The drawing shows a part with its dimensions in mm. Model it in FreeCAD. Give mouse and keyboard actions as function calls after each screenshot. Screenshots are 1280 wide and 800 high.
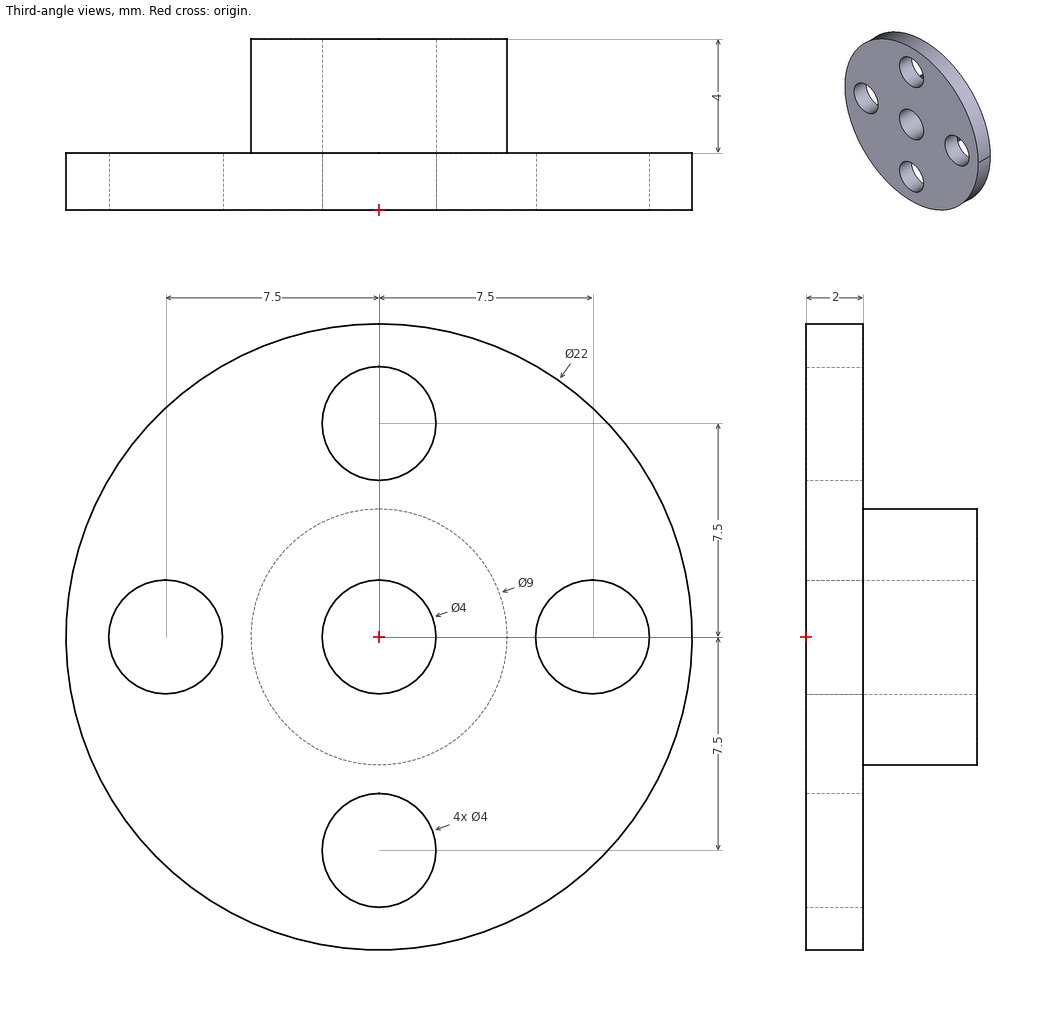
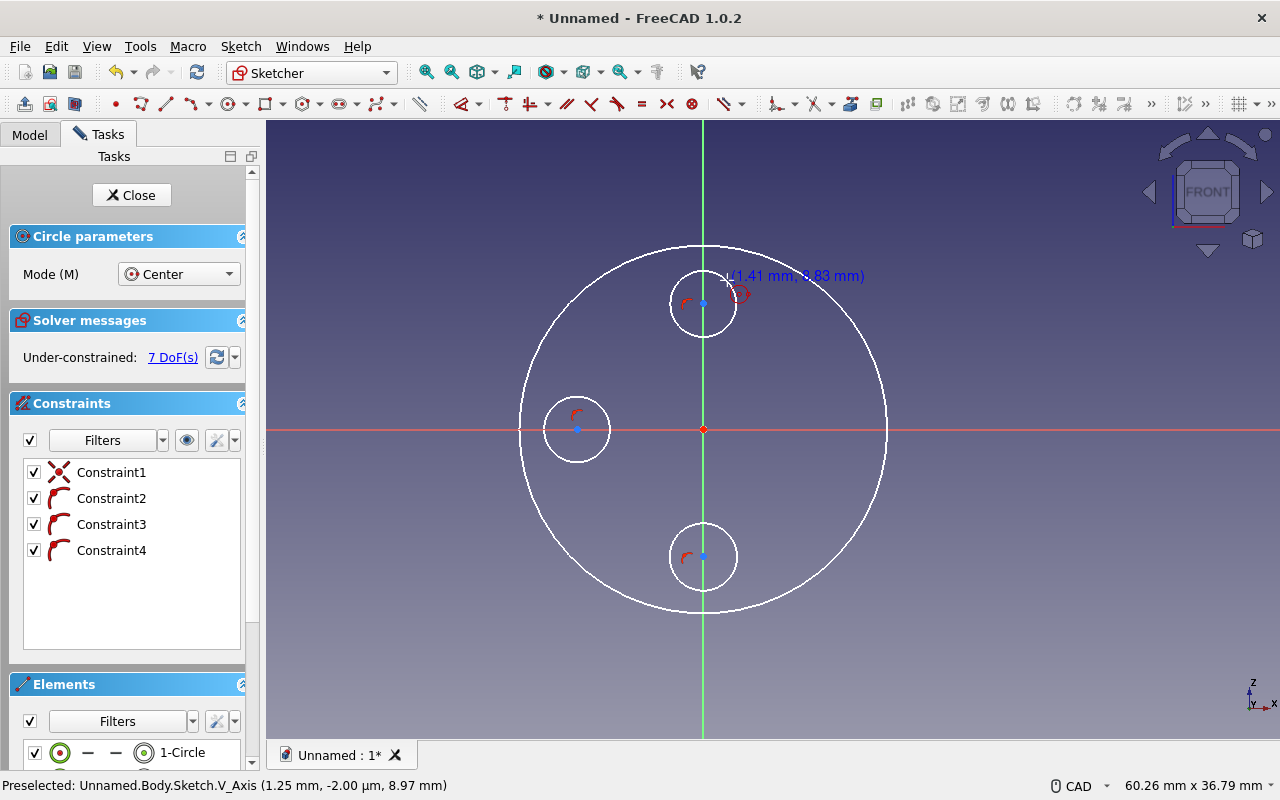
click(830, 430)
click(853, 406)
key(Escape)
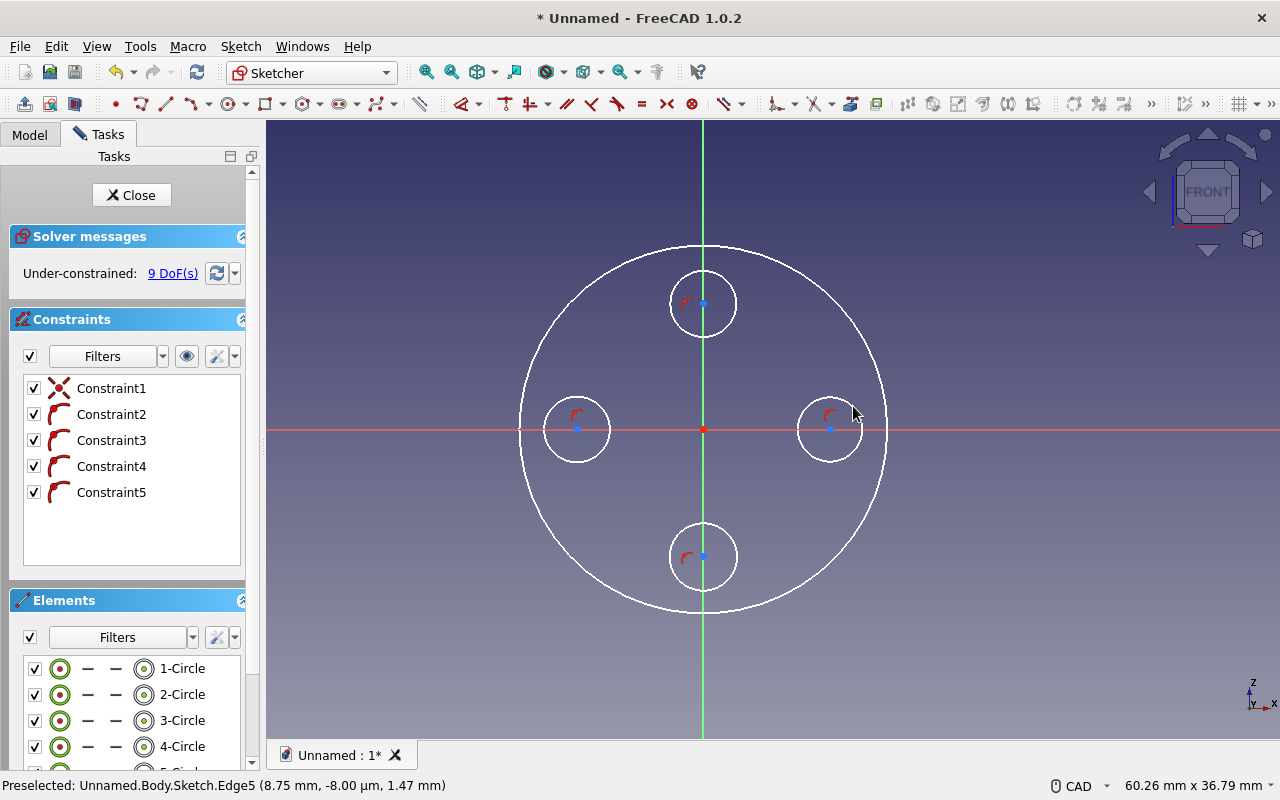
click(727, 533)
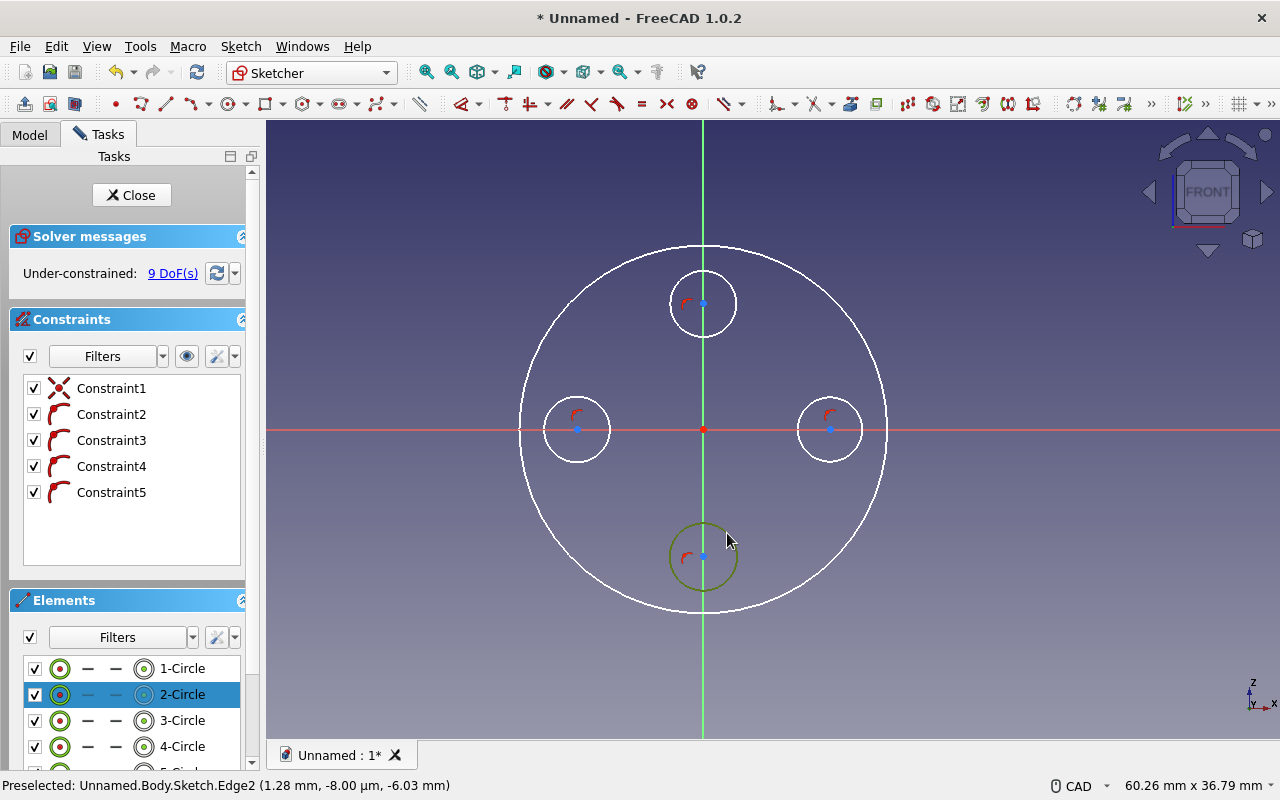
click(600, 406)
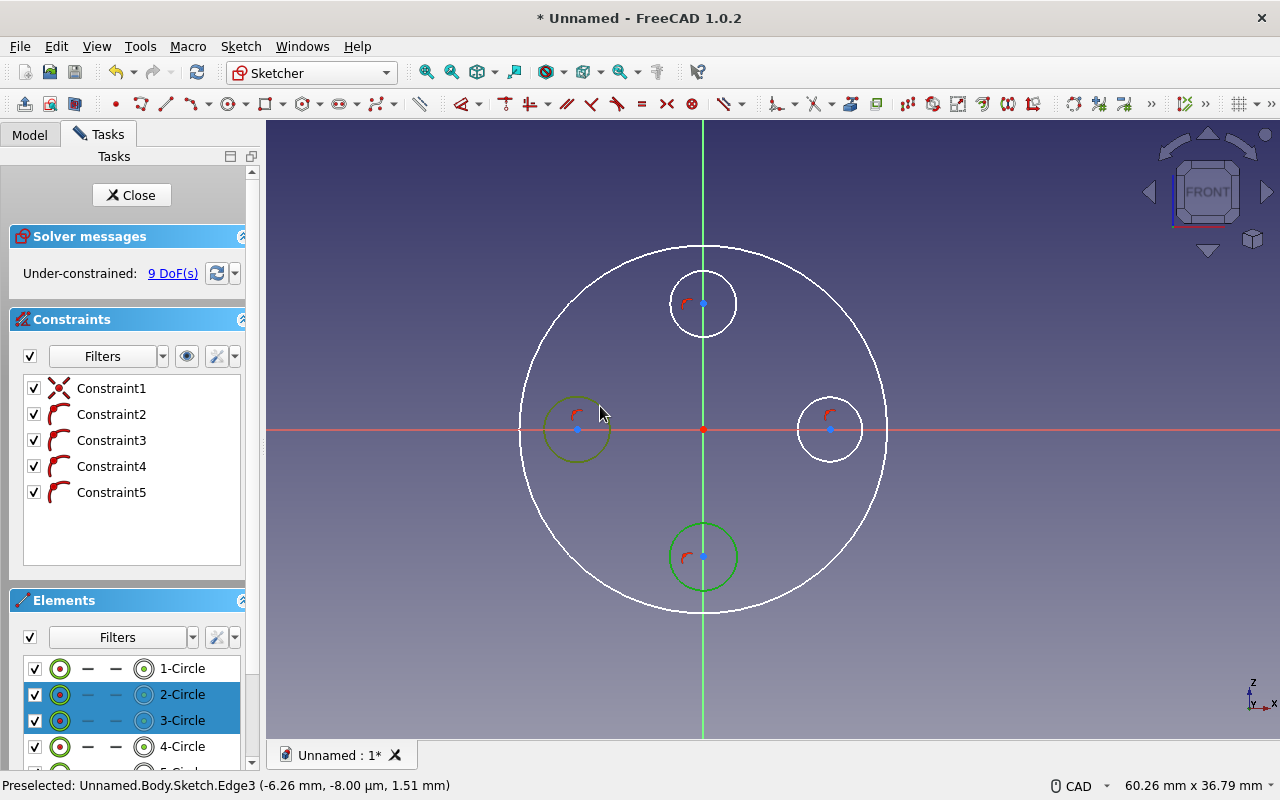
click(727, 281)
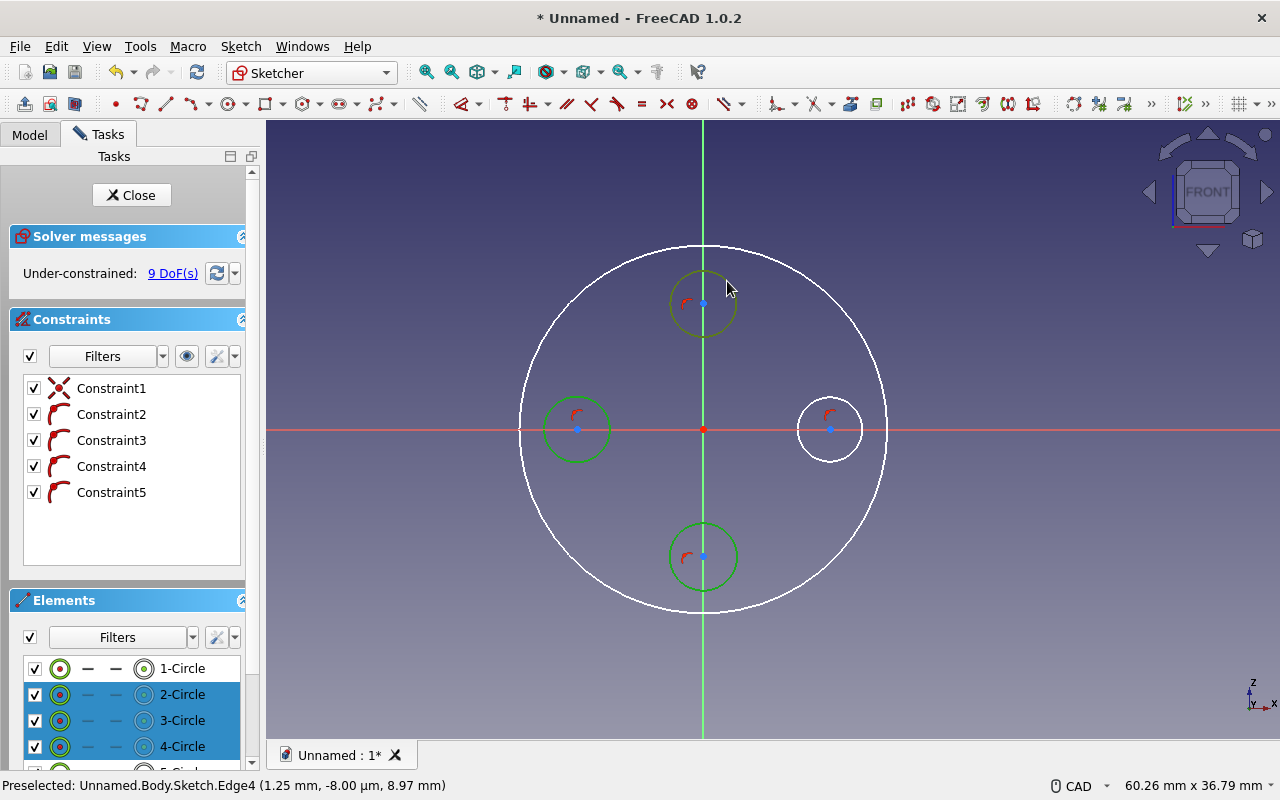
click(853, 407)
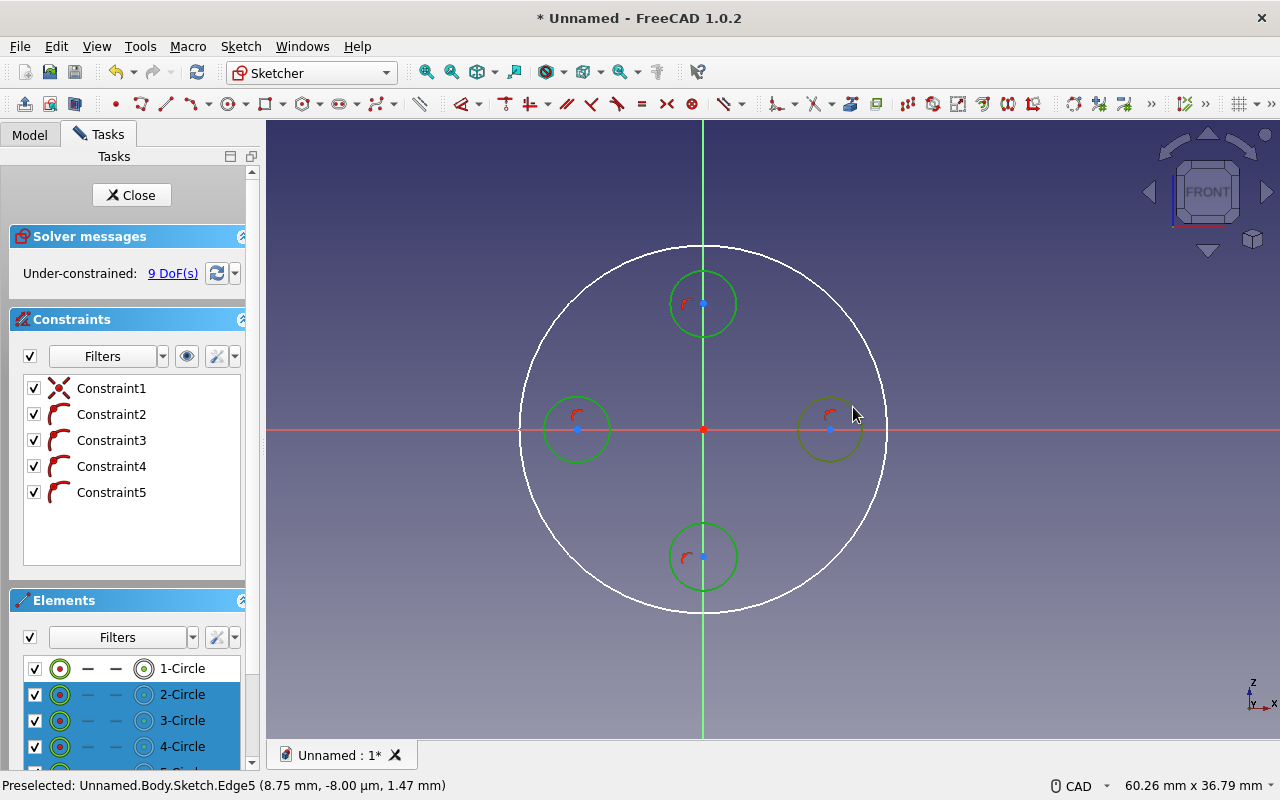
click(642, 104)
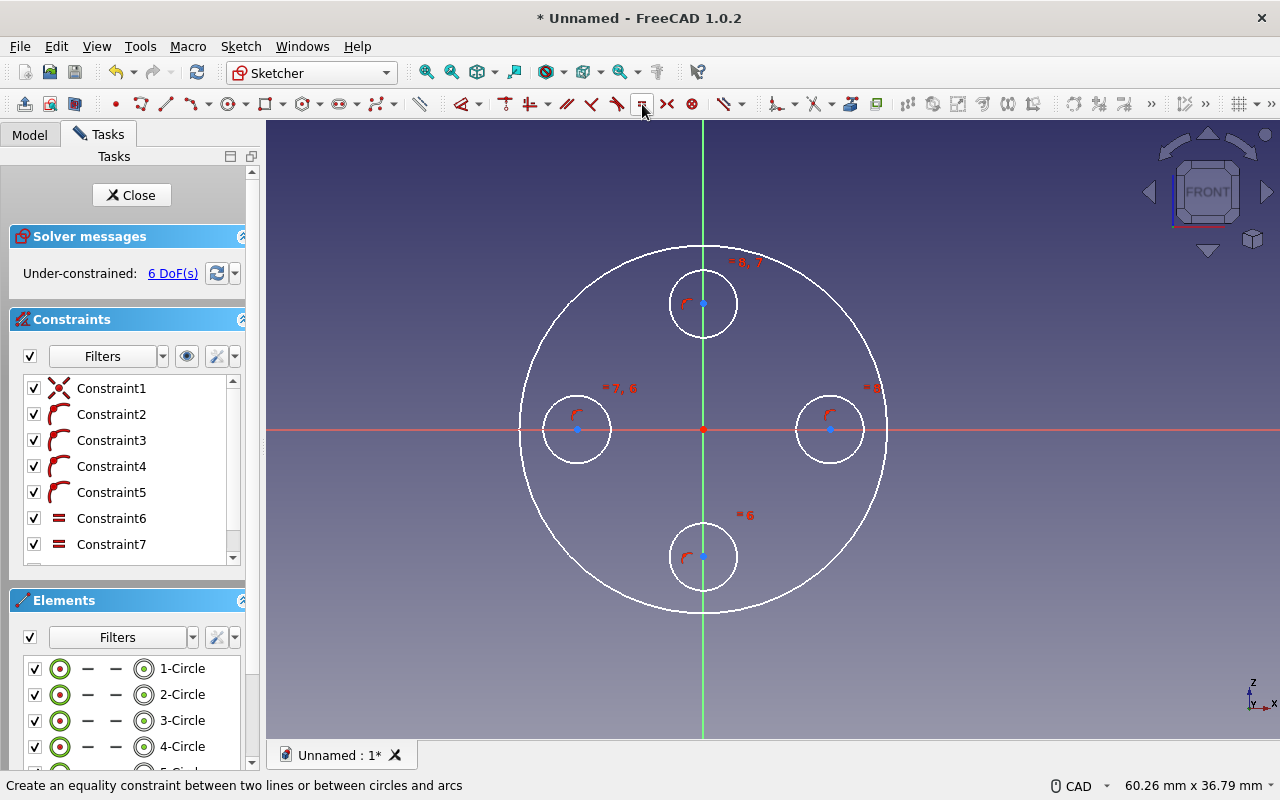
click(460, 104)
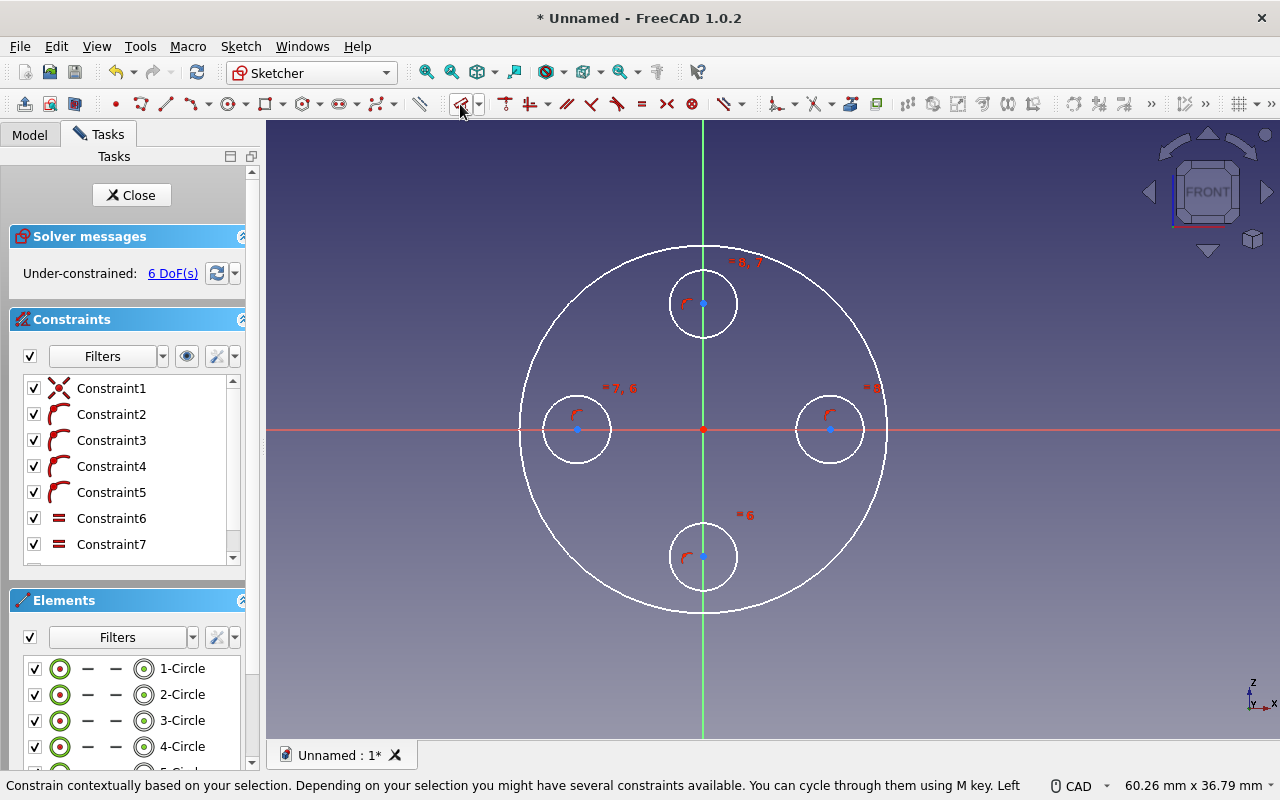
click(833, 299)
click(856, 276)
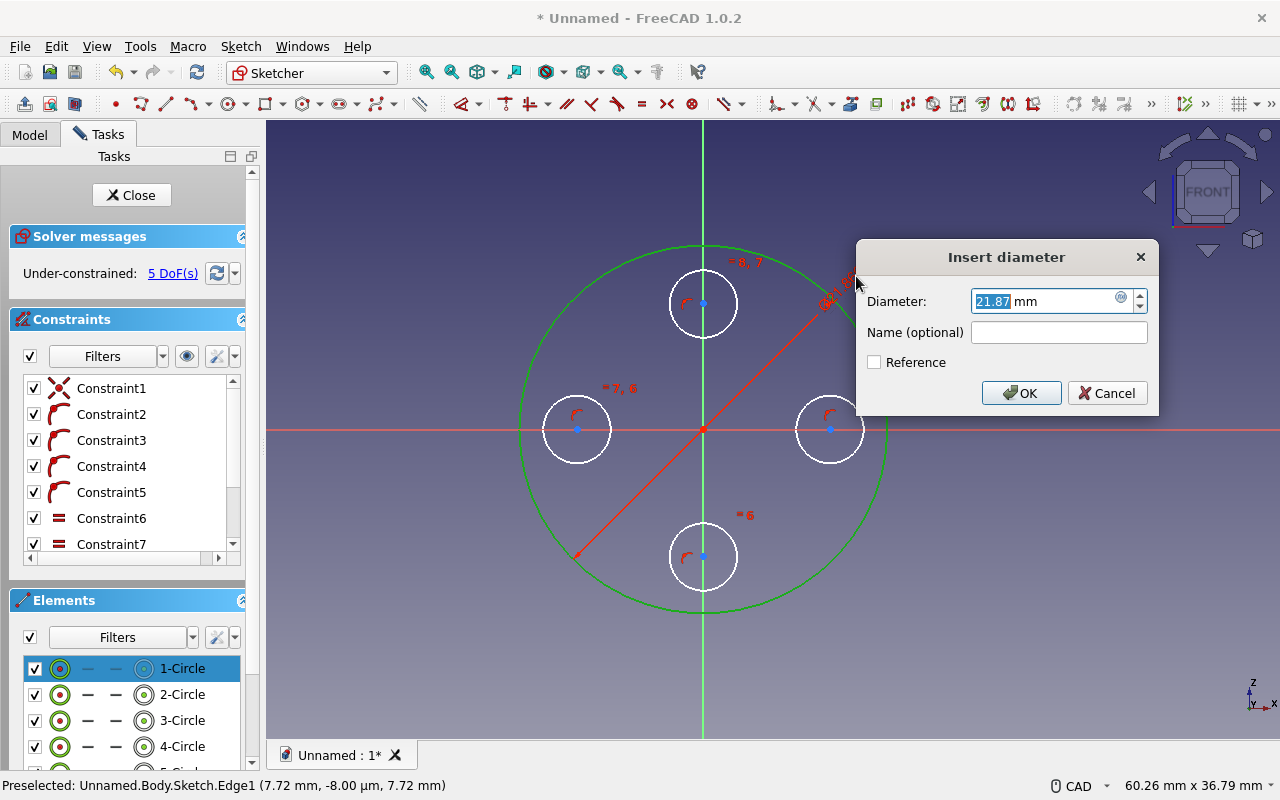
text(22)
key(Return)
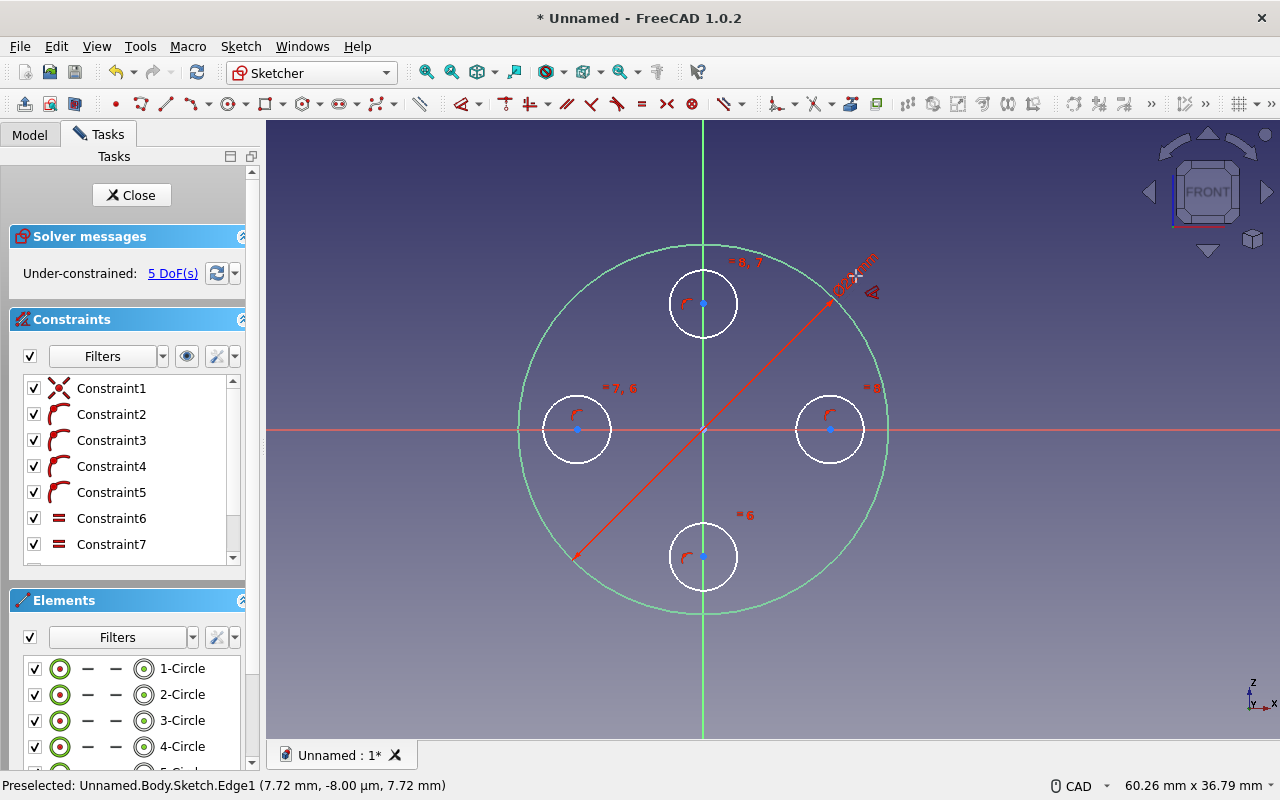
click(727, 533)
click(749, 510)